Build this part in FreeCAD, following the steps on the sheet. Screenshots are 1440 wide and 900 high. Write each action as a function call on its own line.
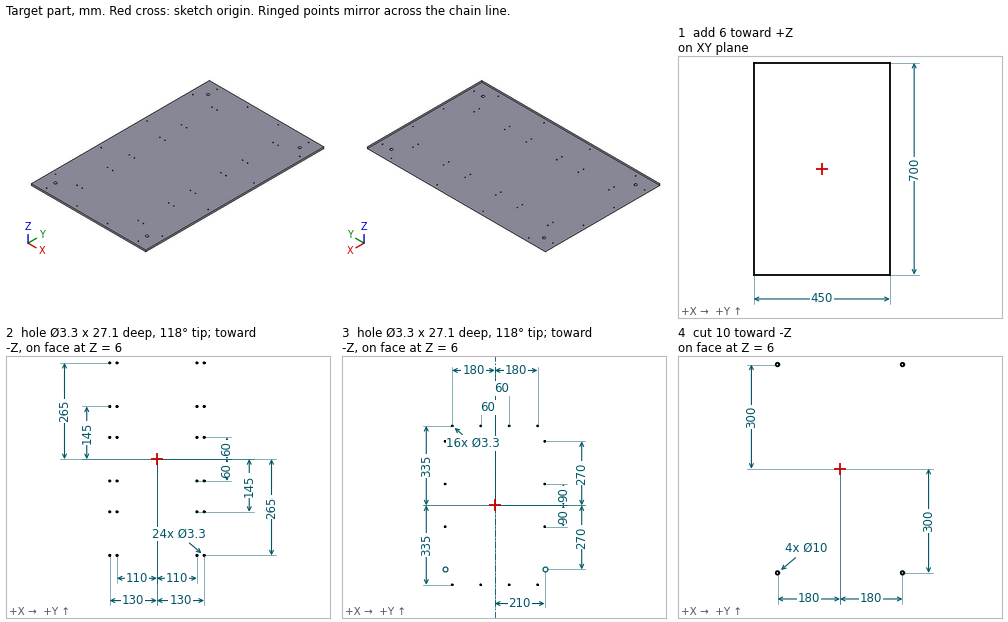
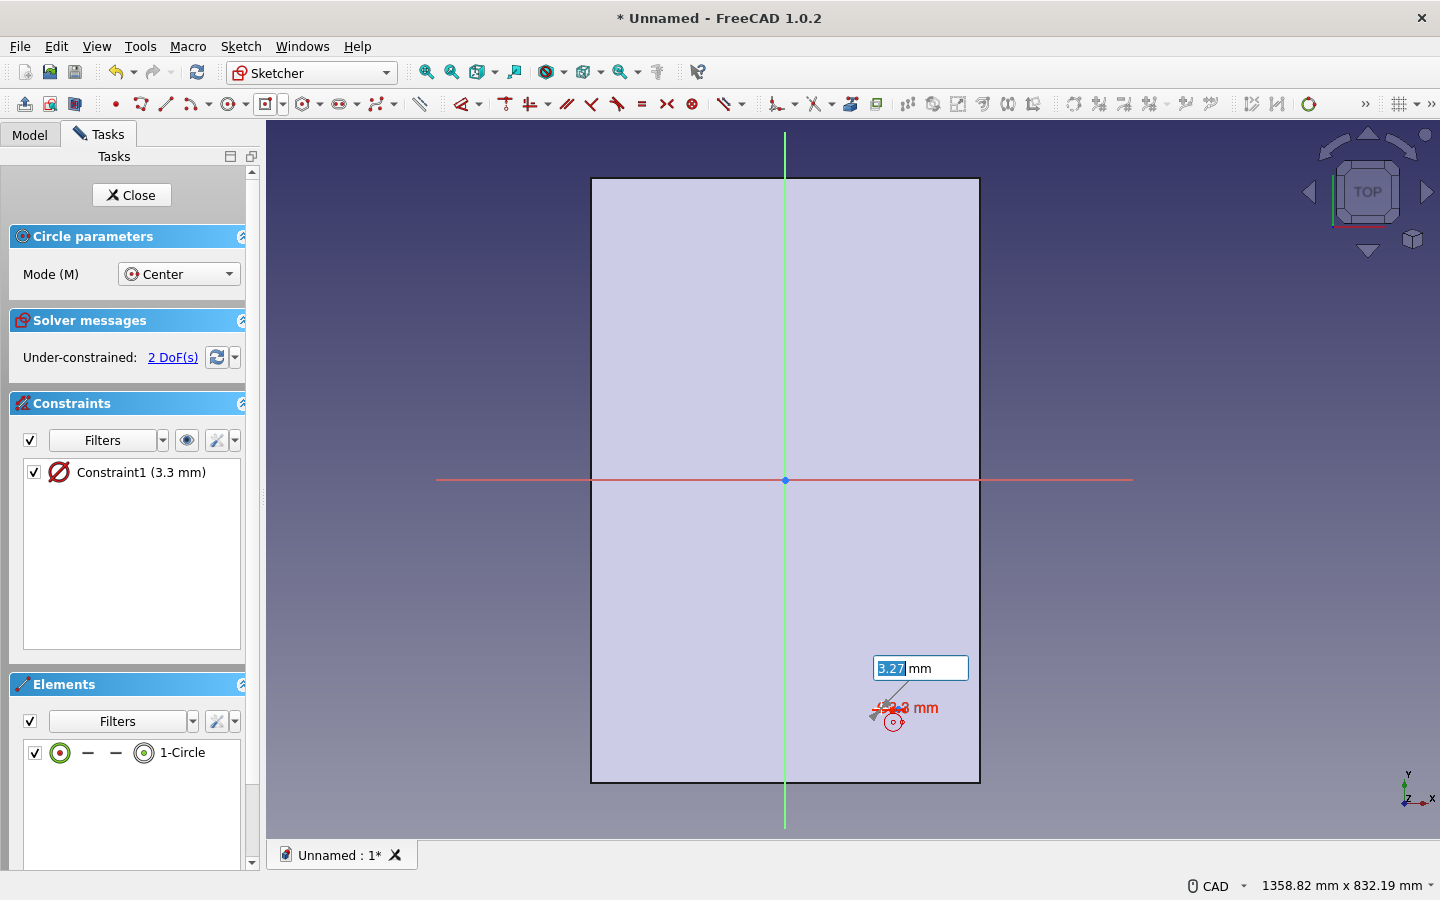
text(3.3)
key(Return)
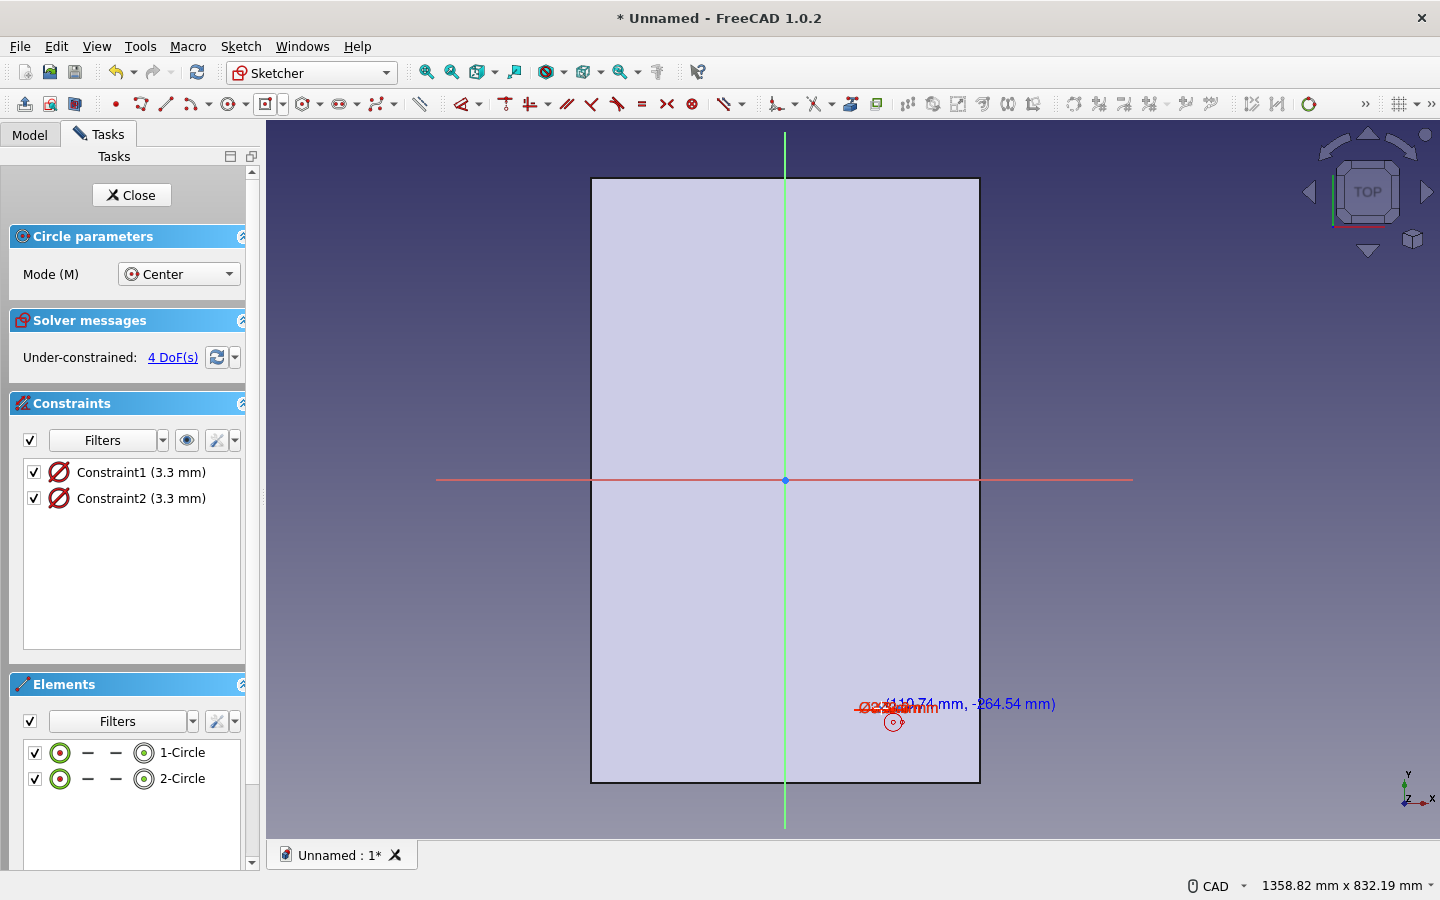
scroll(880, 606, up, 14)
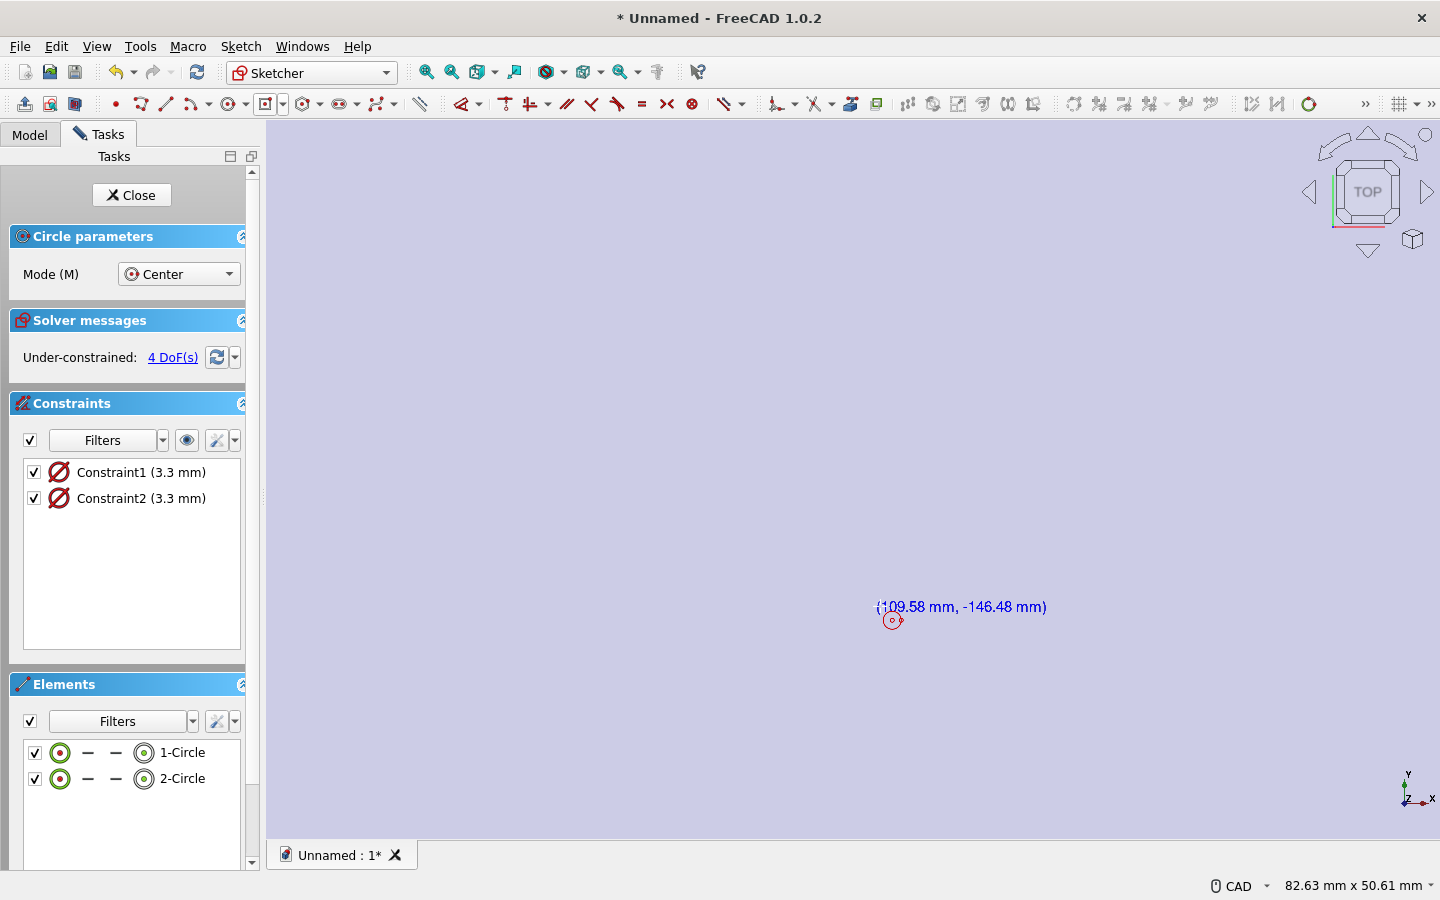
scroll(880, 606, down, 14)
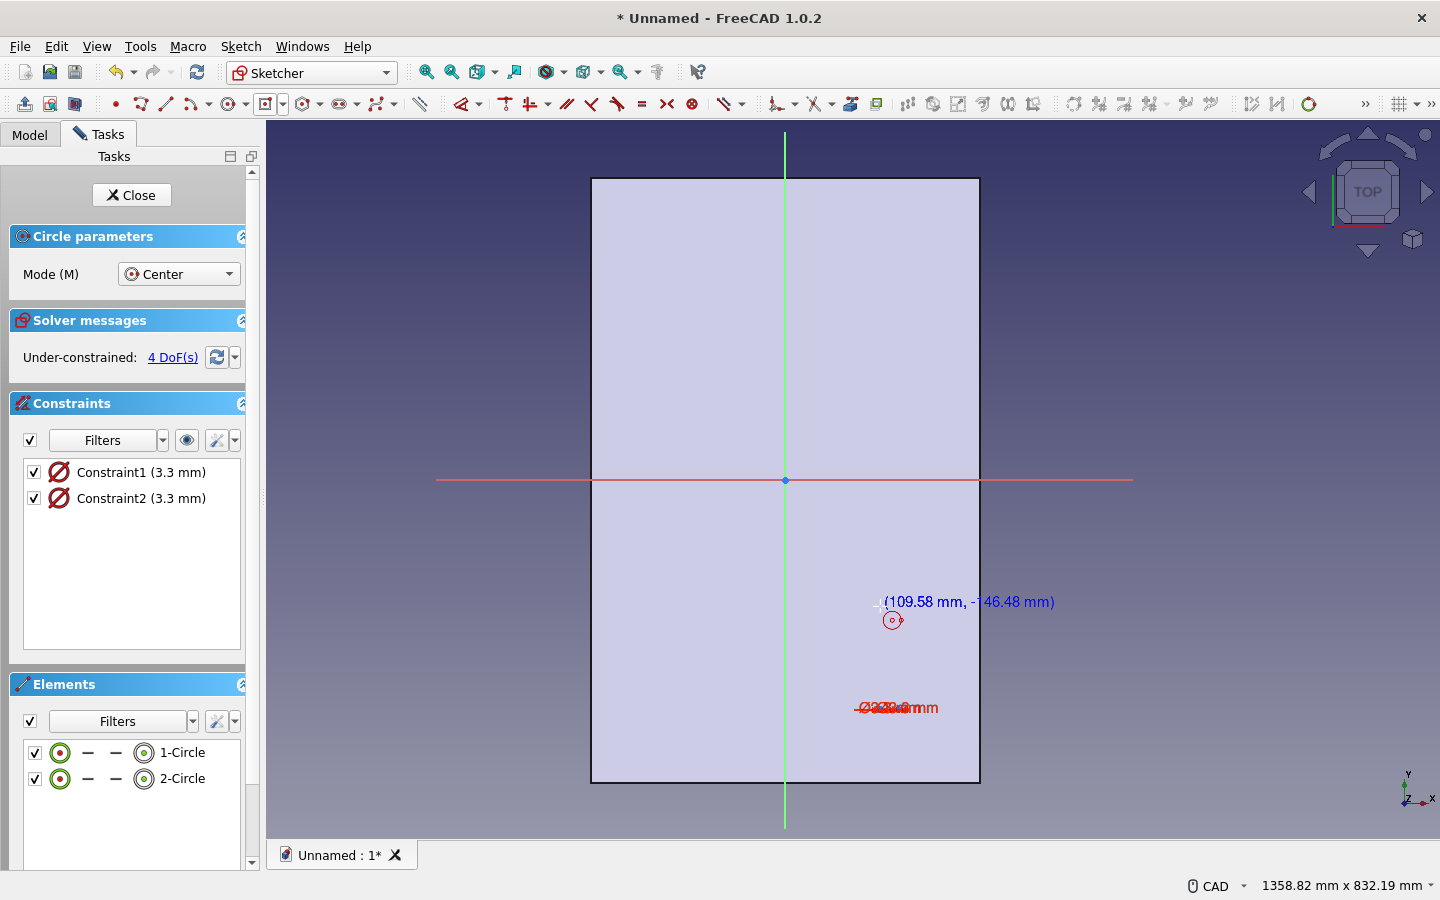
click(880, 606)
move(881, 605)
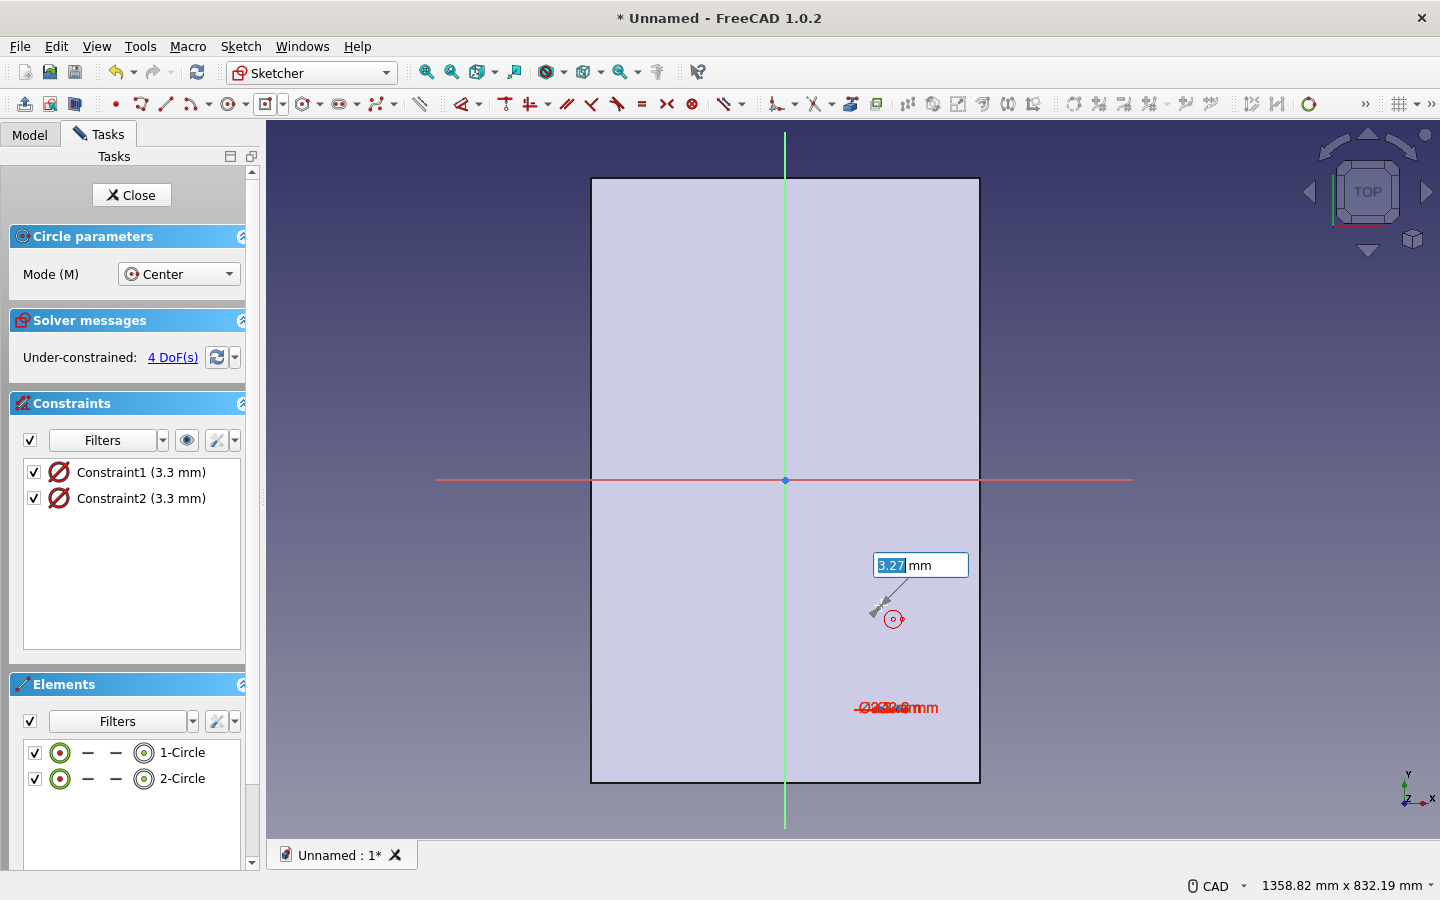
text(3.3)
key(Return)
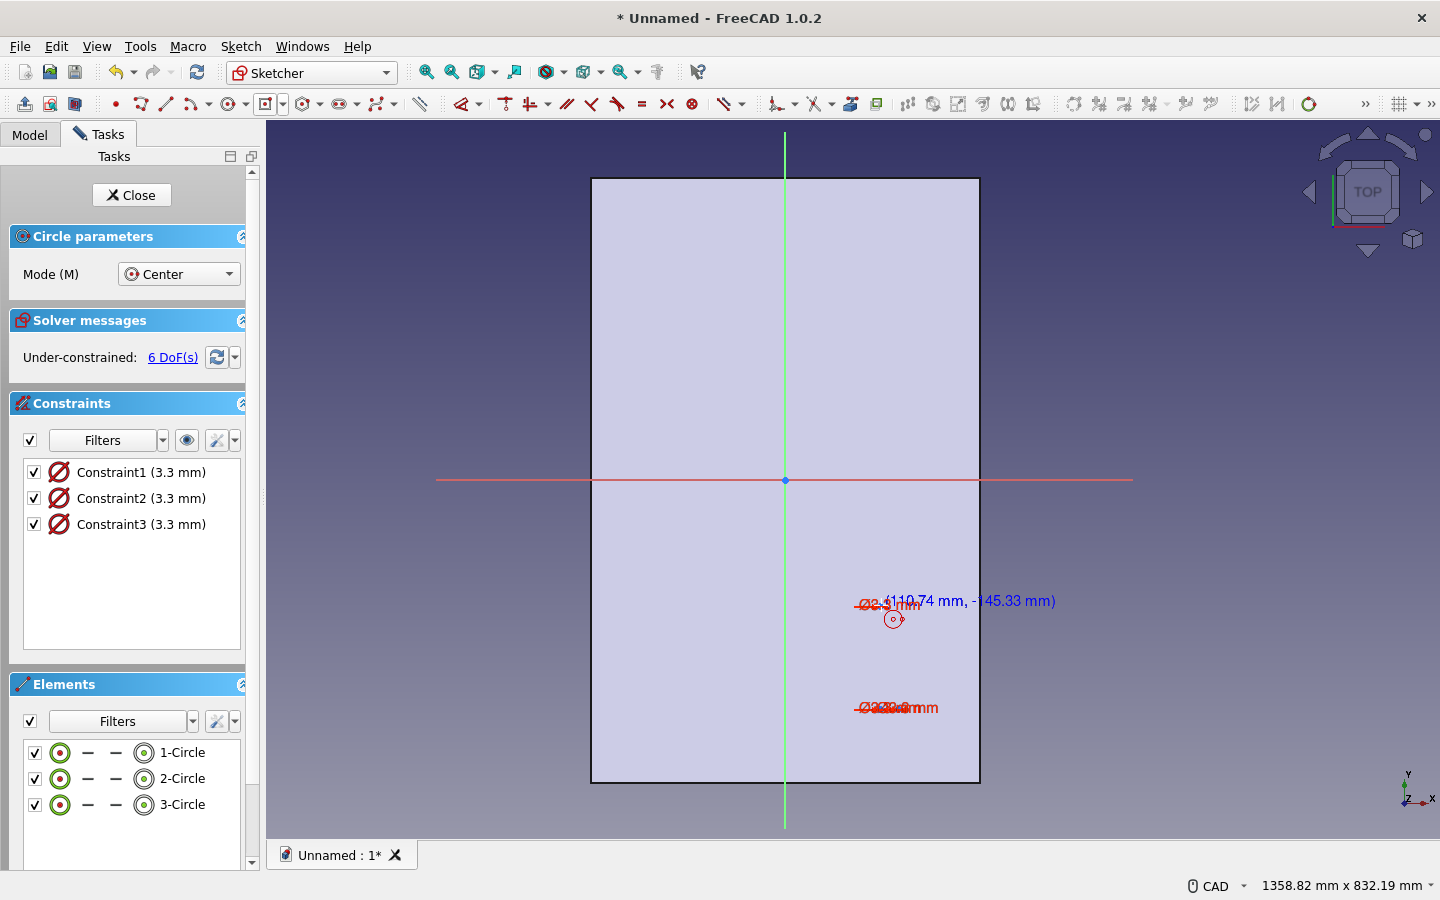
scroll(898, 606, up, 14)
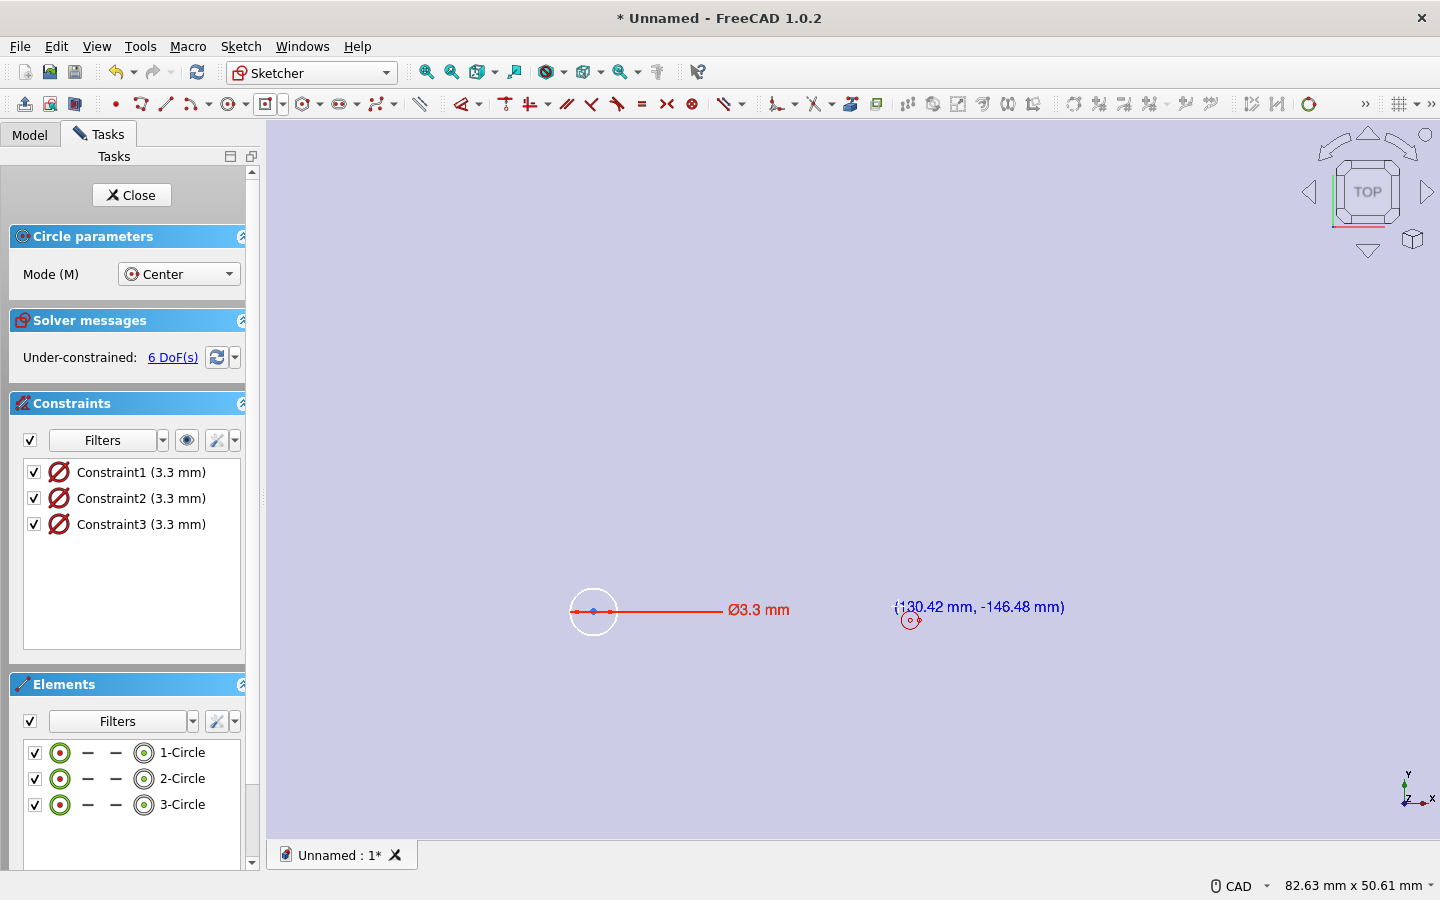
scroll(898, 606, down, 14)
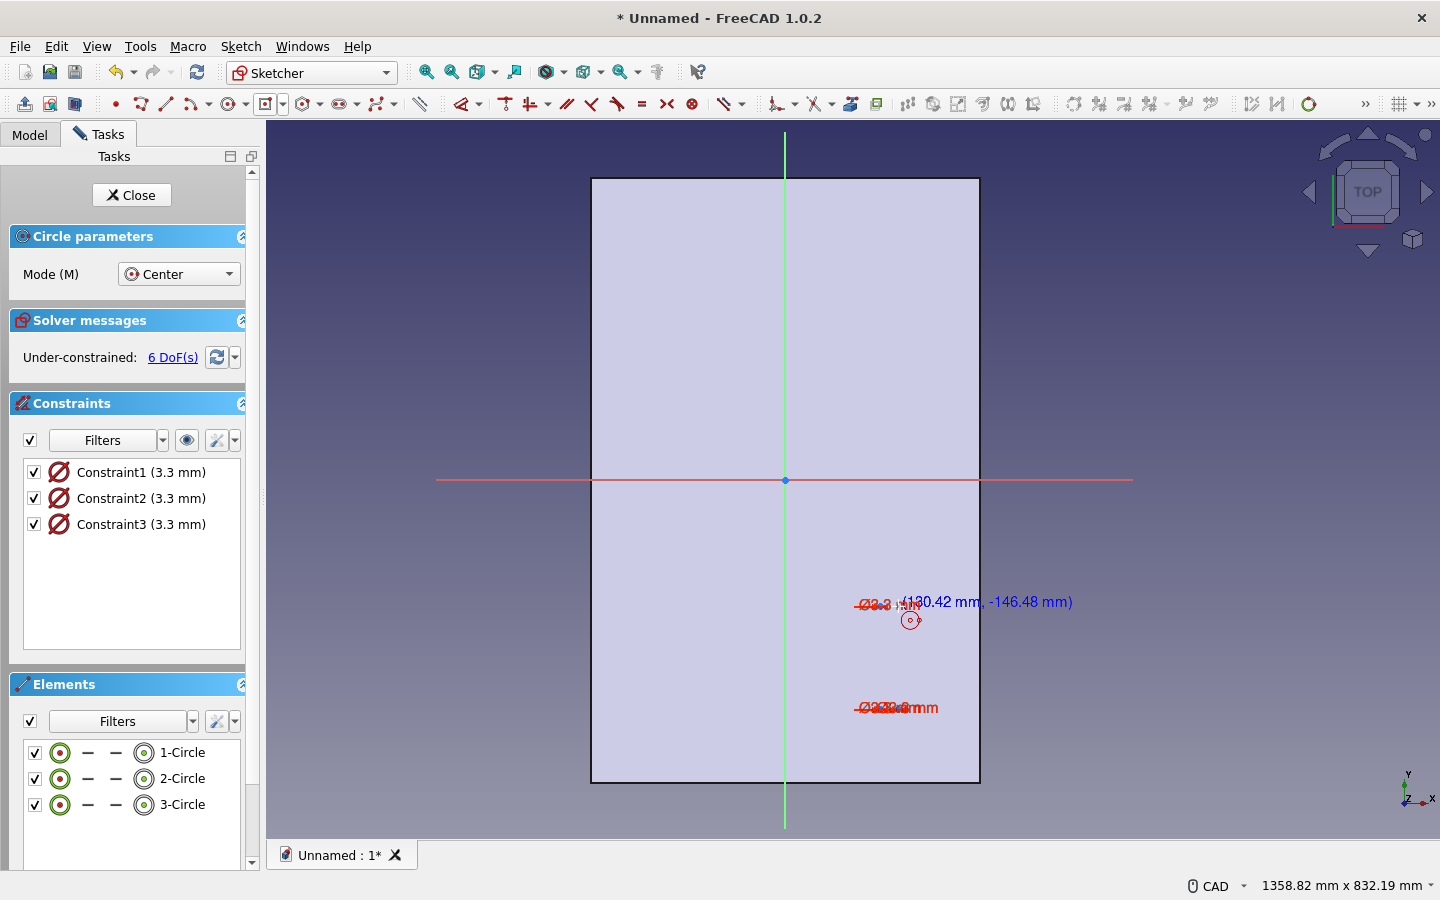
click(898, 606)
move(899, 605)